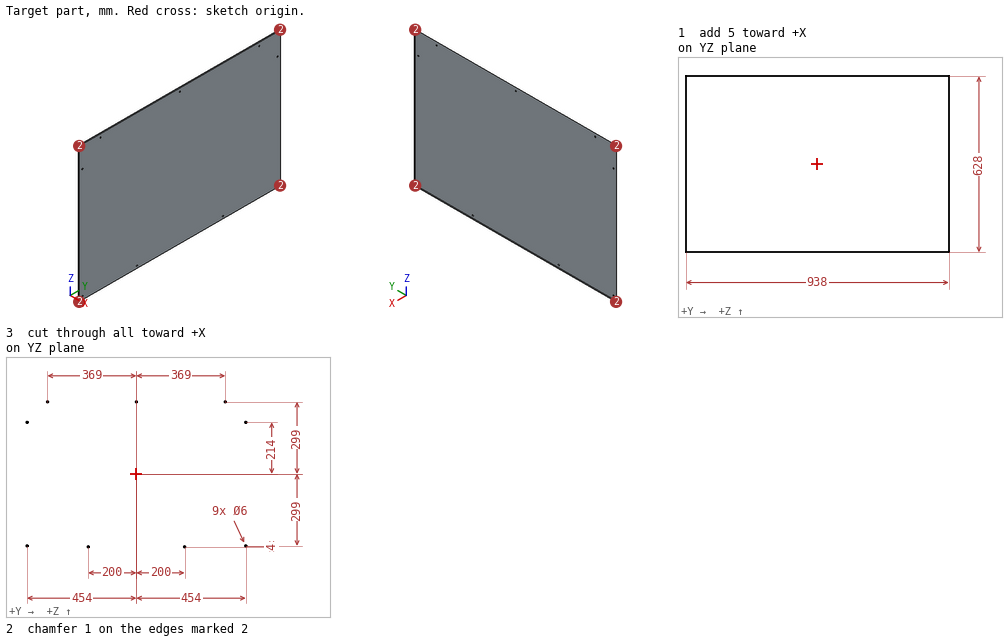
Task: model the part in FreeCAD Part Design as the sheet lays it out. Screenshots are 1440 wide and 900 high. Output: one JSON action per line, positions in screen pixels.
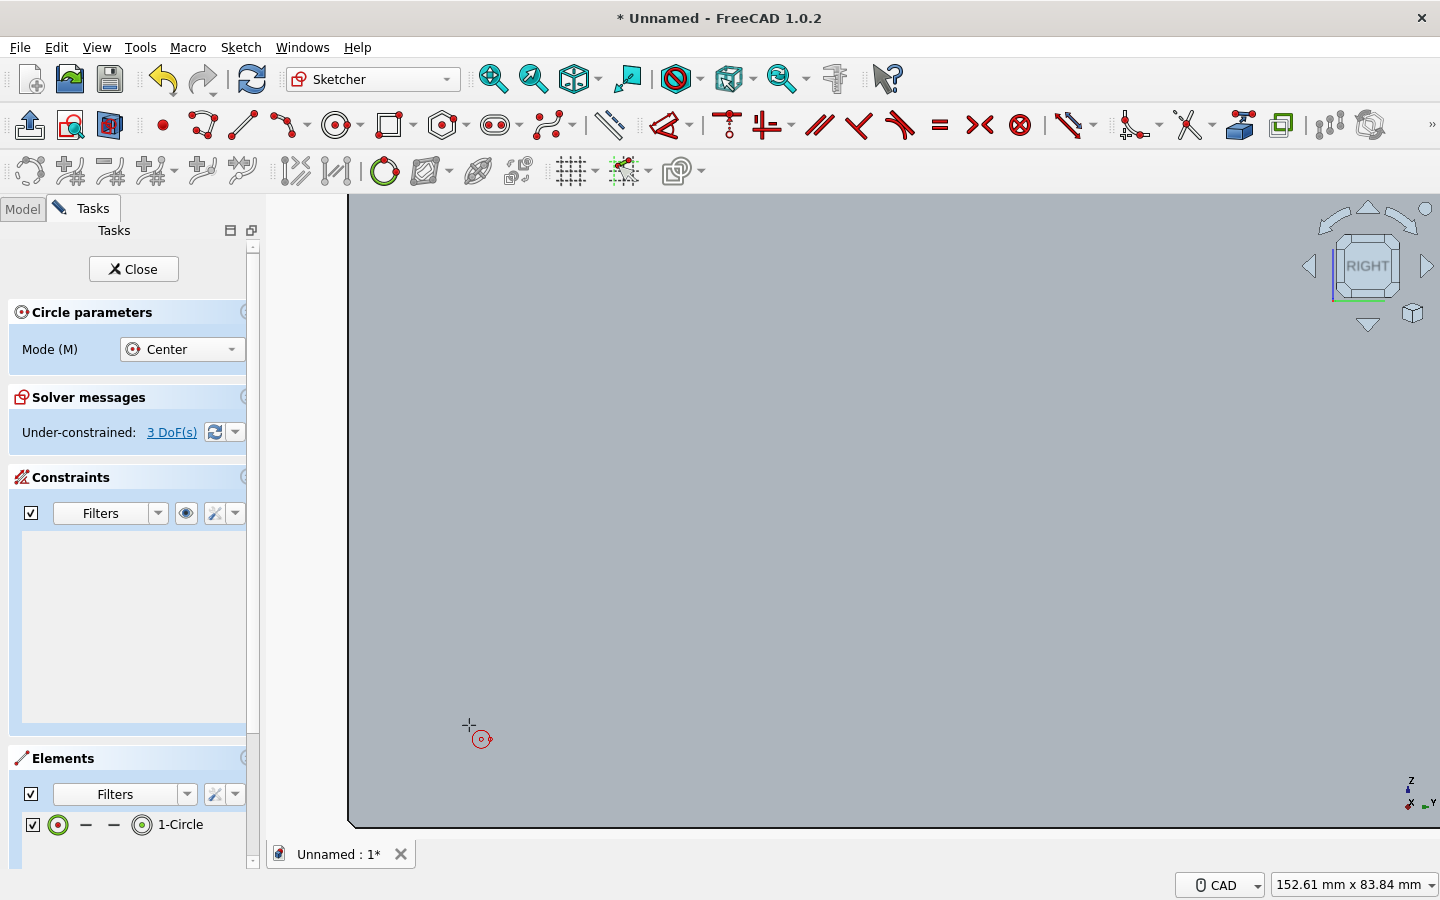
{"action": "scroll", "coordinate": [468, 725], "scroll_direction": "down", "scroll_amount": 12}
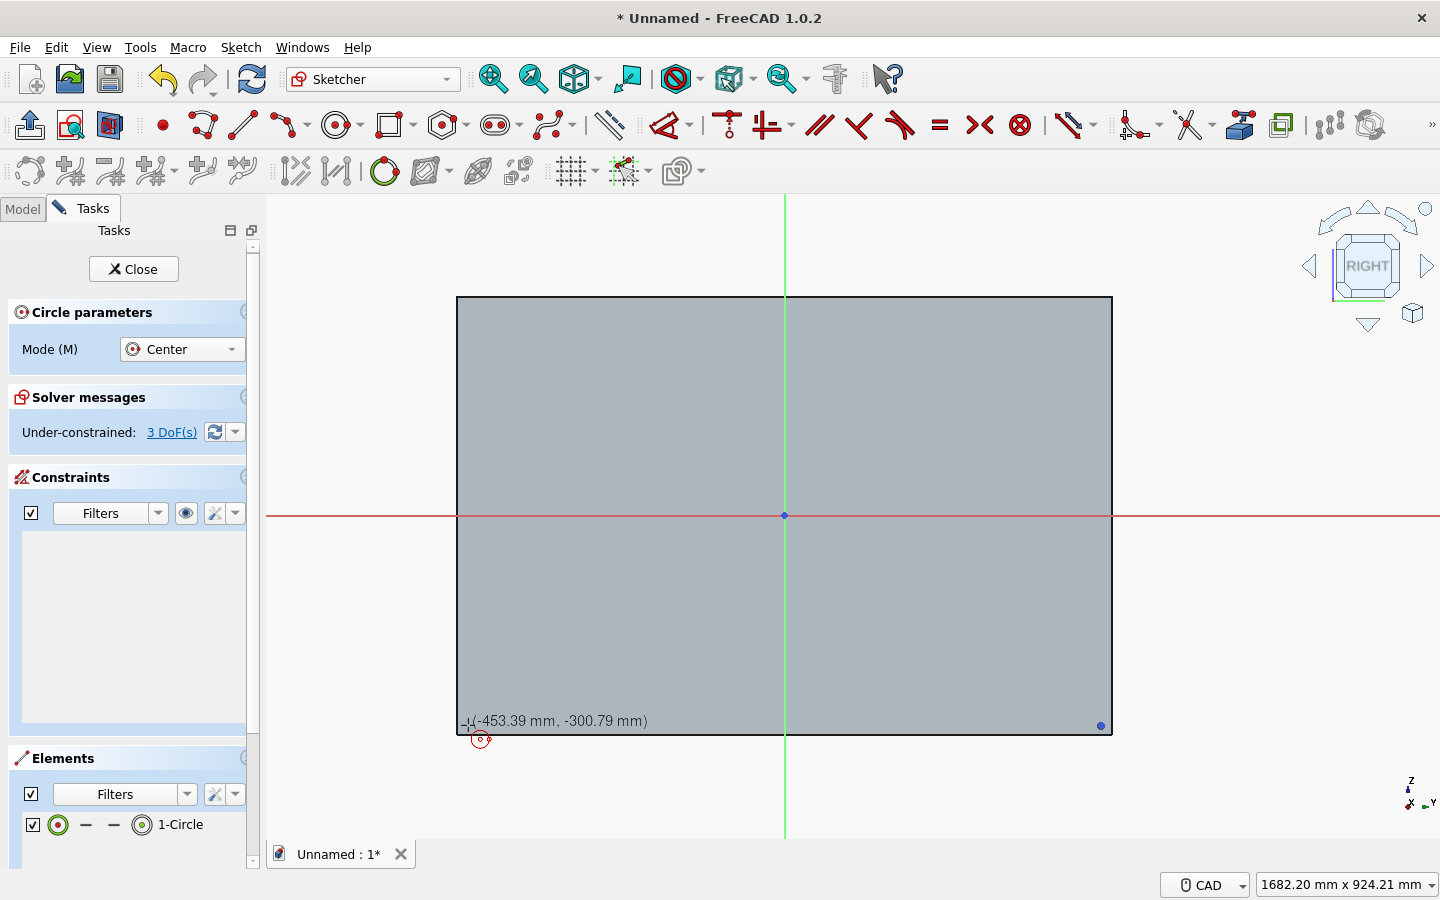
{"action": "left_click", "coordinate": [468, 725]}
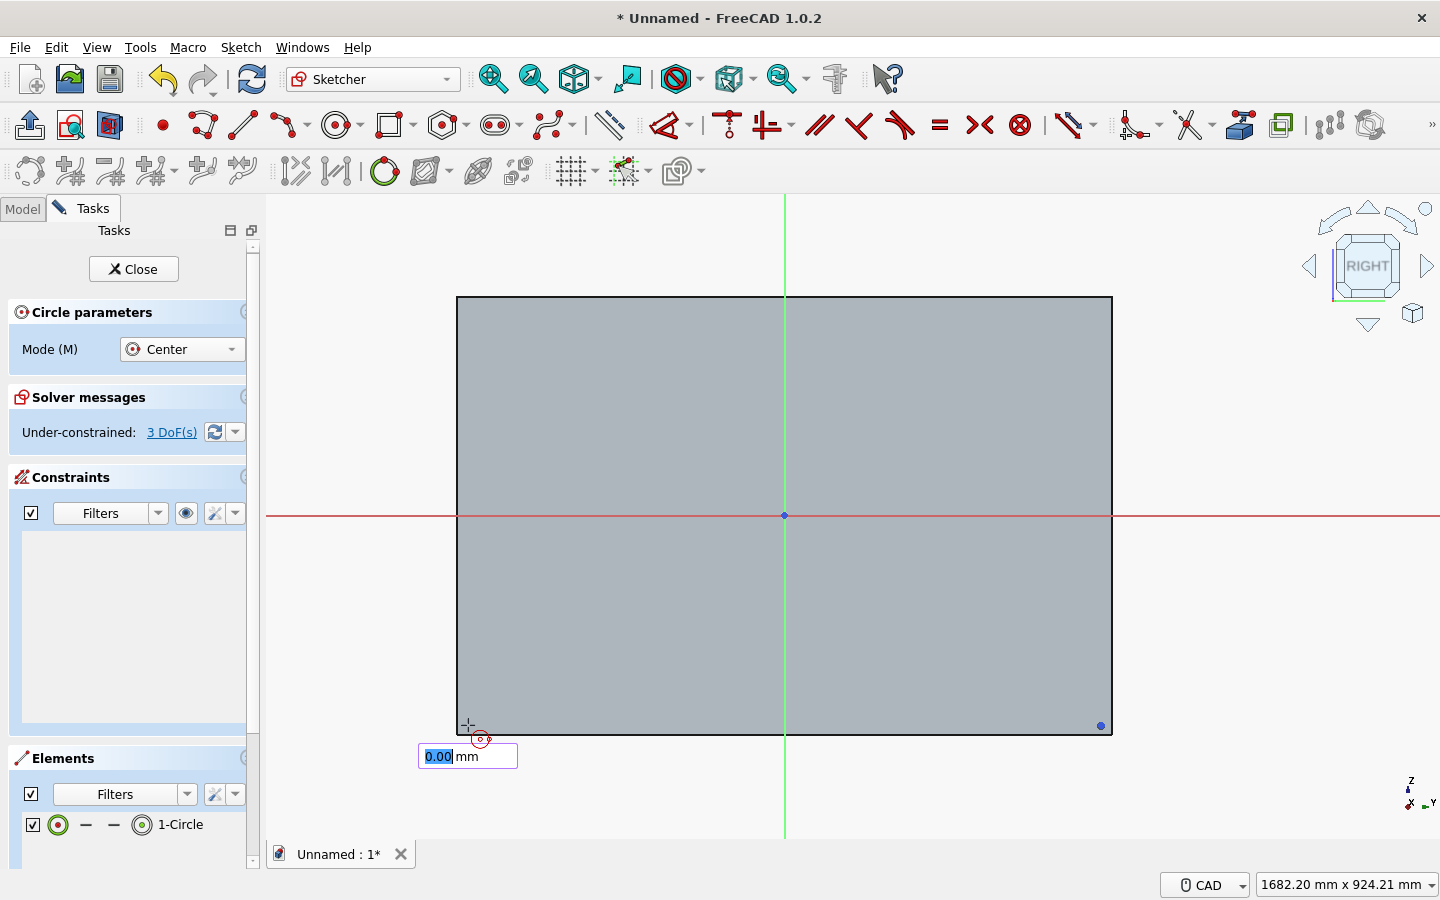
{"action": "scroll", "coordinate": [469, 723], "scroll_direction": "up", "scroll_amount": 11}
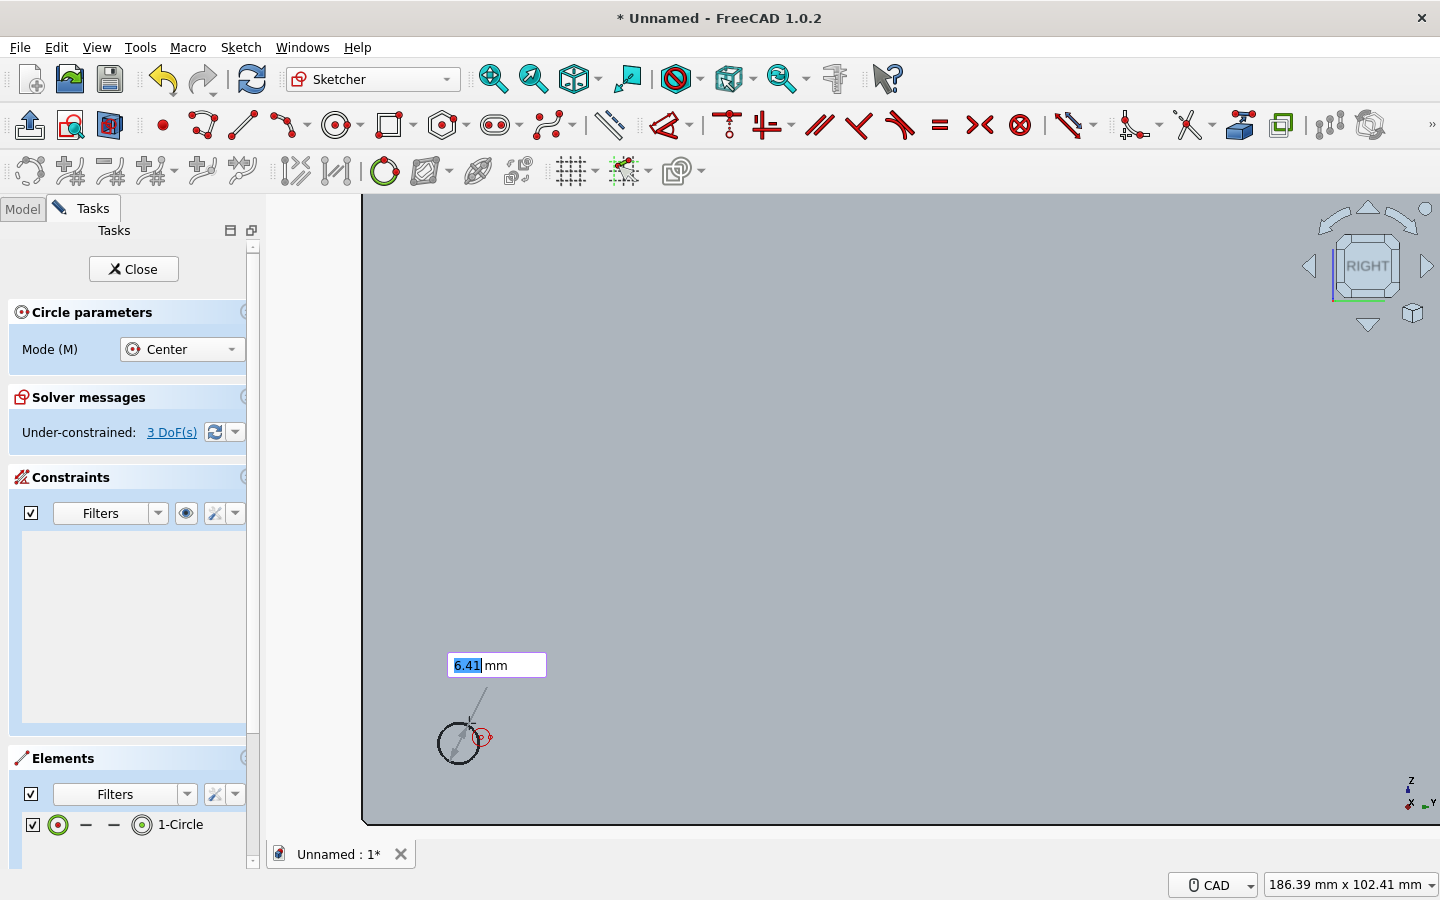
{"action": "left_click", "coordinate": [470, 717]}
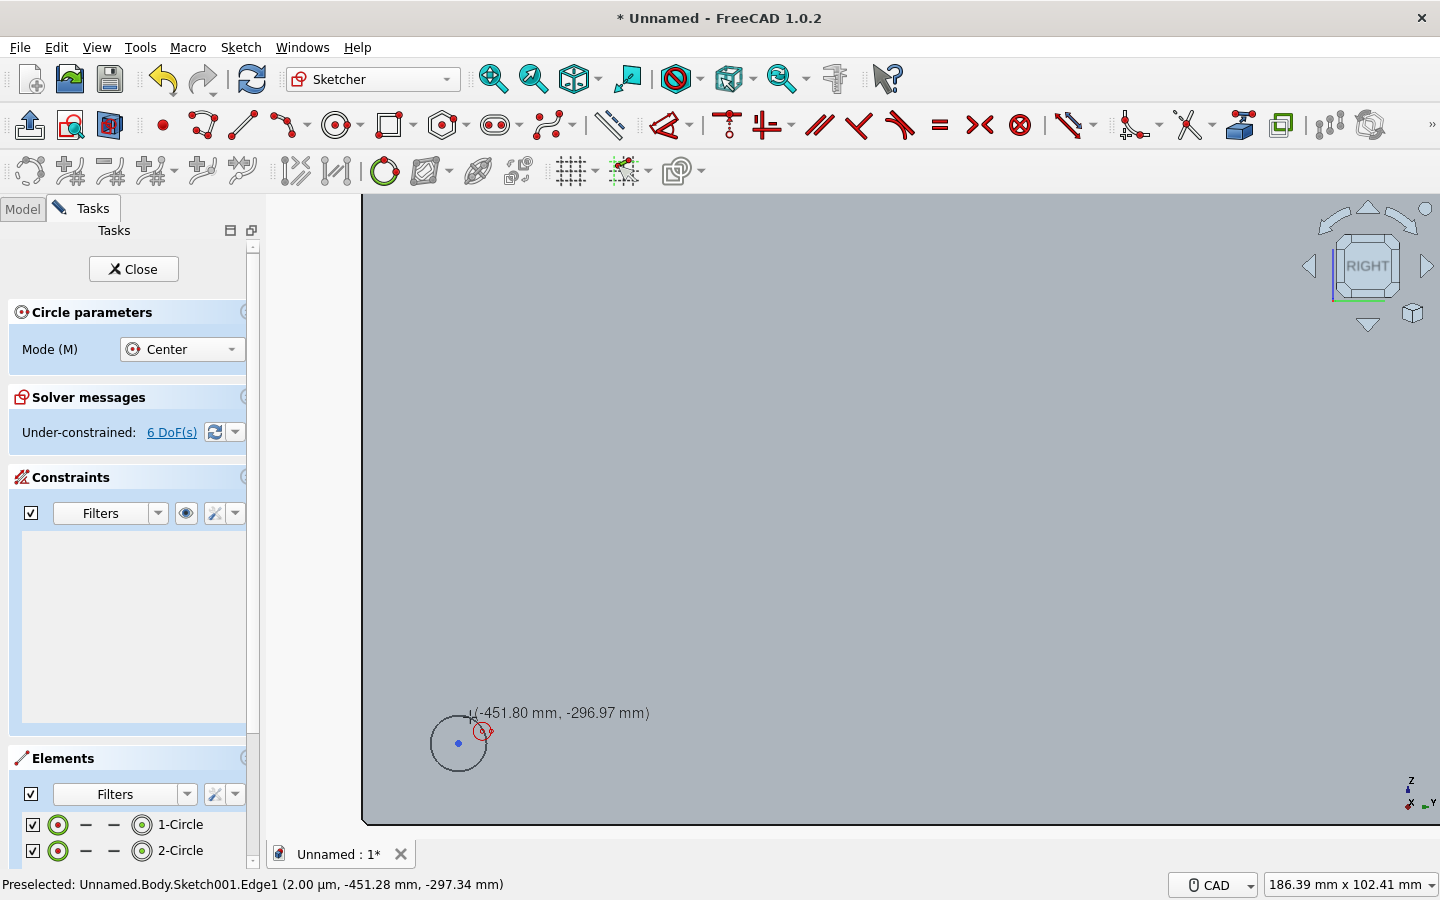
{"action": "scroll", "coordinate": [469, 723], "scroll_direction": "down", "scroll_amount": 11}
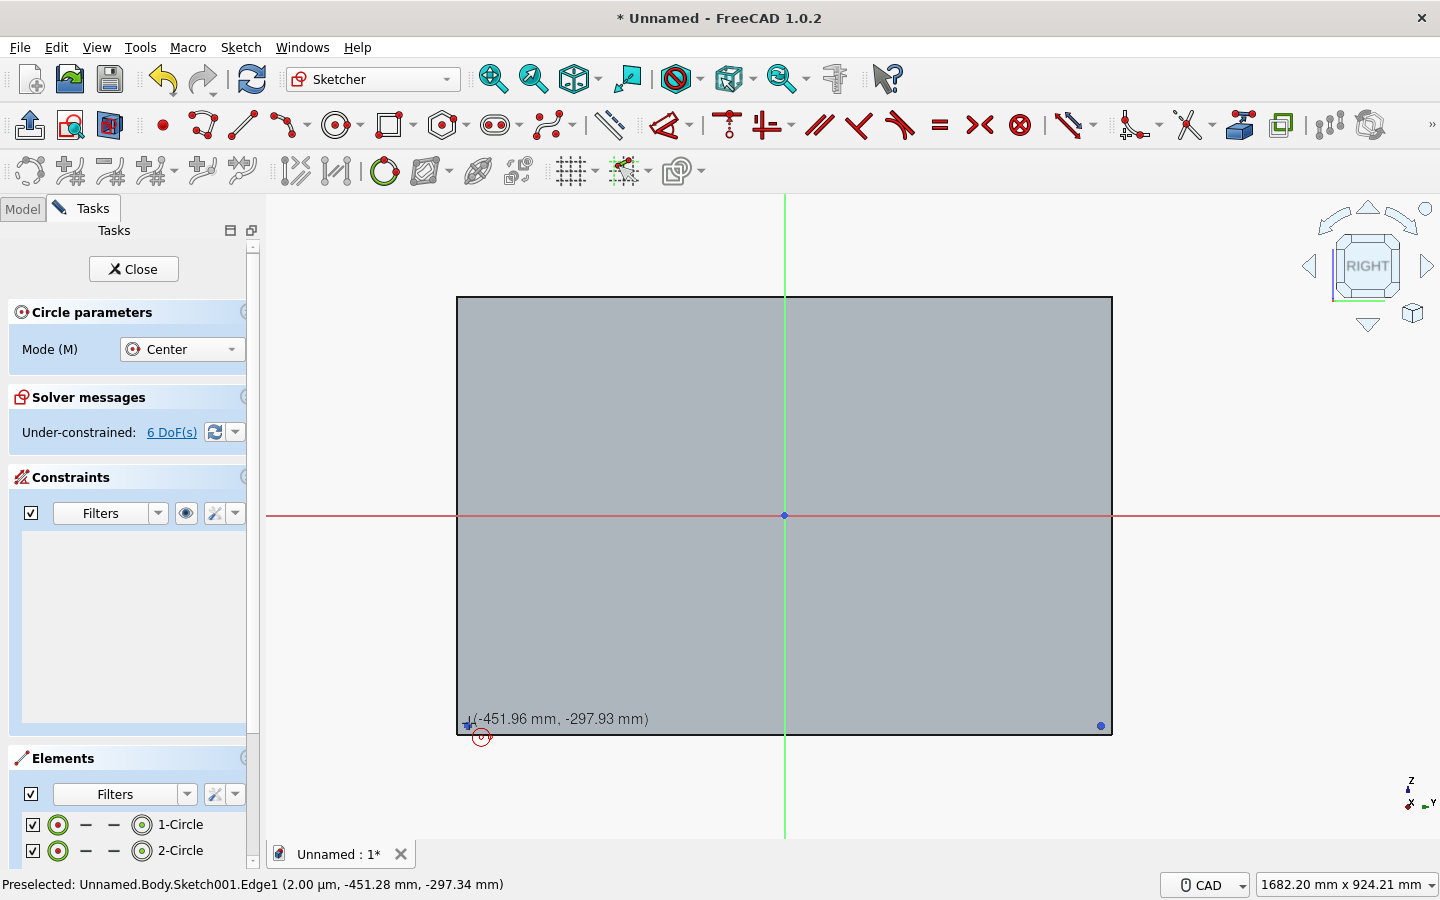
{"action": "scroll", "coordinate": [1101, 367], "scroll_direction": "up", "scroll_amount": 12}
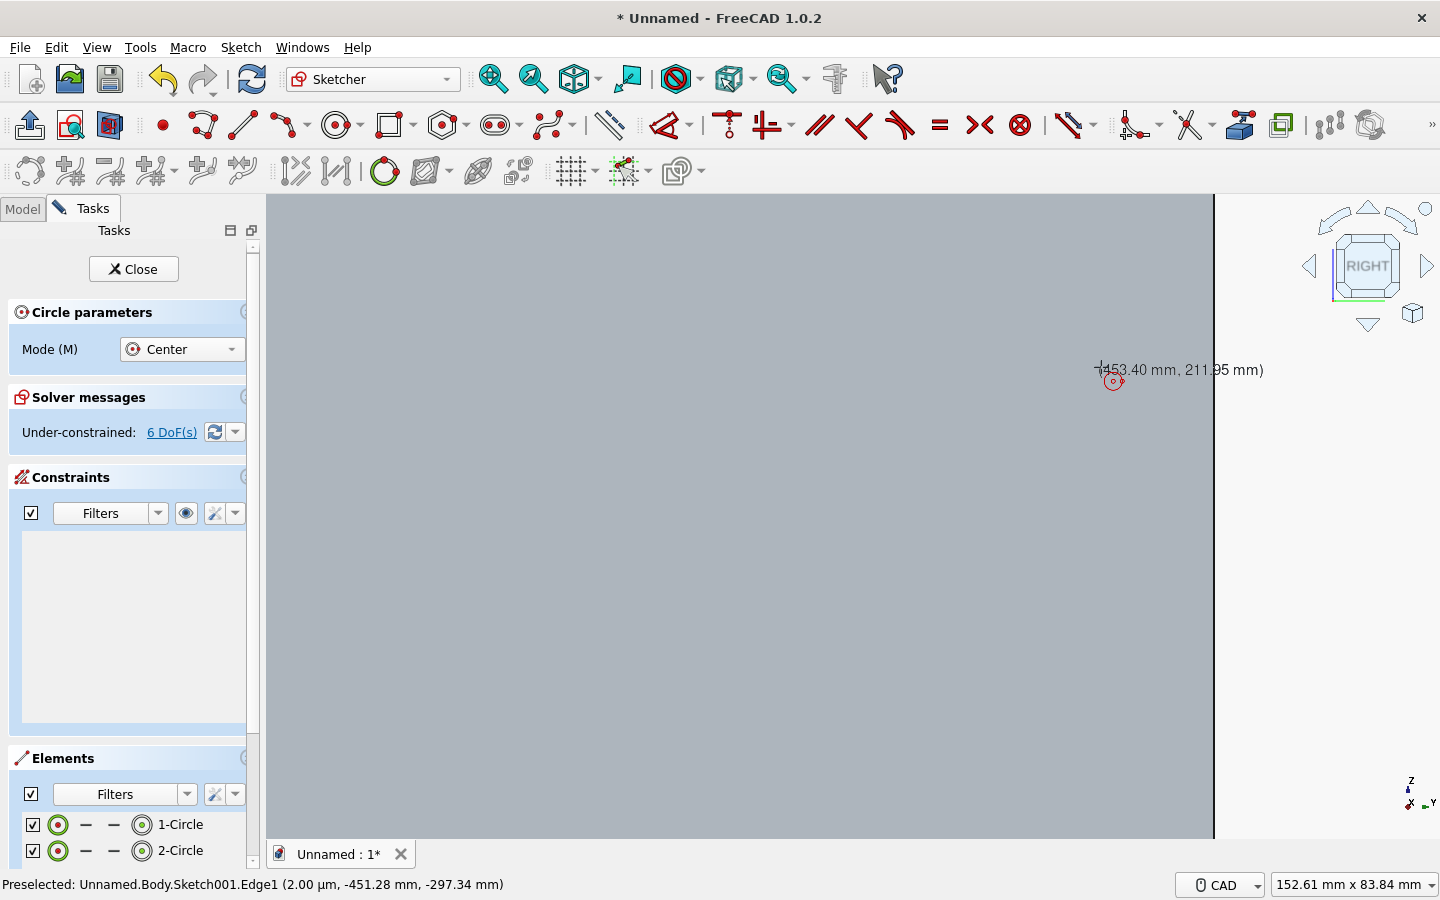
{"action": "scroll", "coordinate": [1102, 366], "scroll_direction": "down", "scroll_amount": 12}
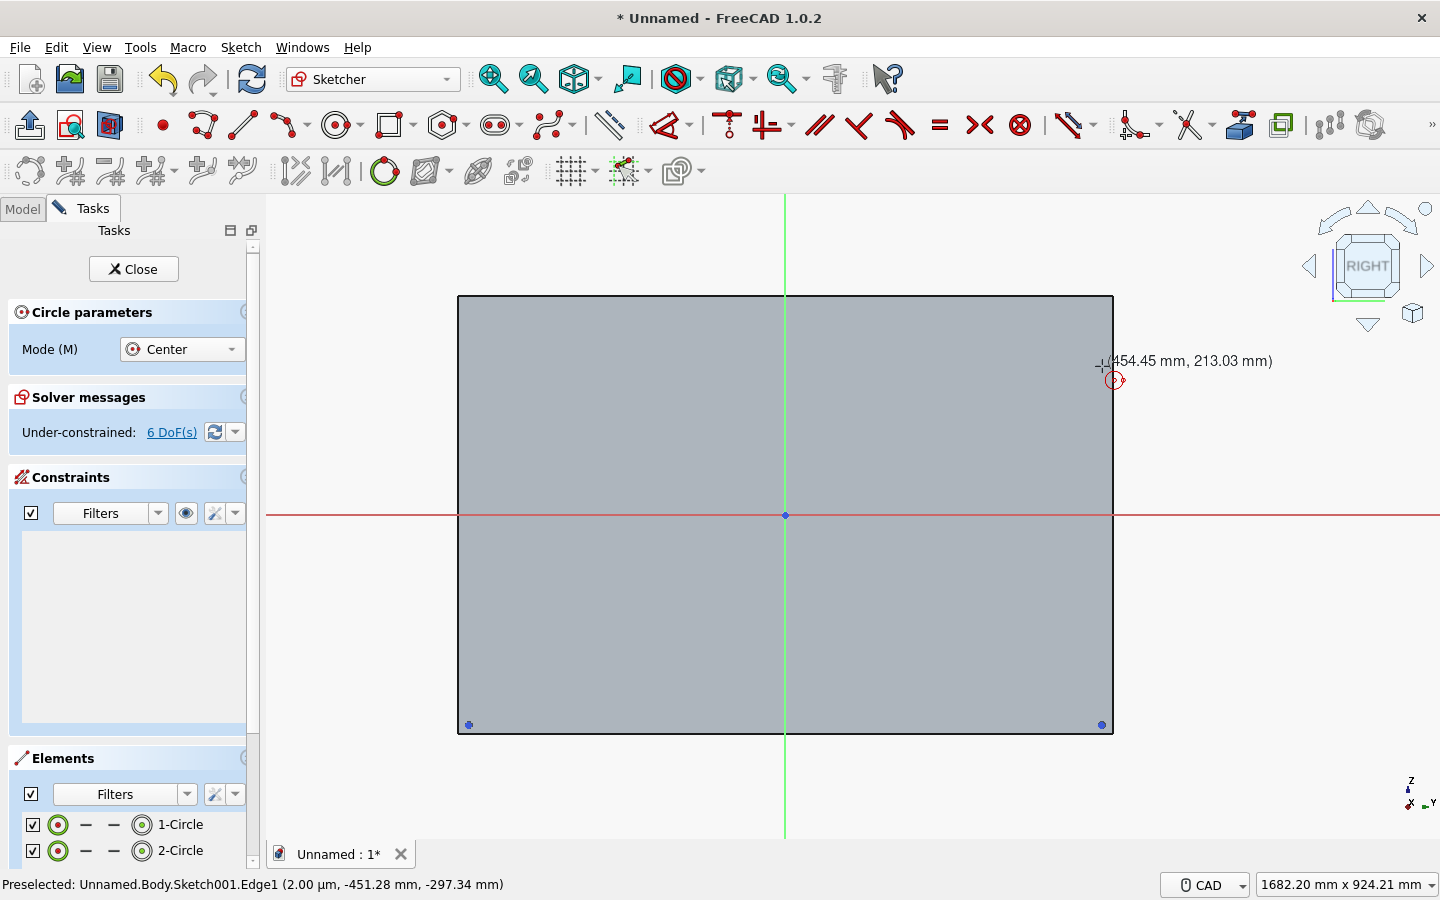
{"action": "left_click", "coordinate": [1102, 366]}